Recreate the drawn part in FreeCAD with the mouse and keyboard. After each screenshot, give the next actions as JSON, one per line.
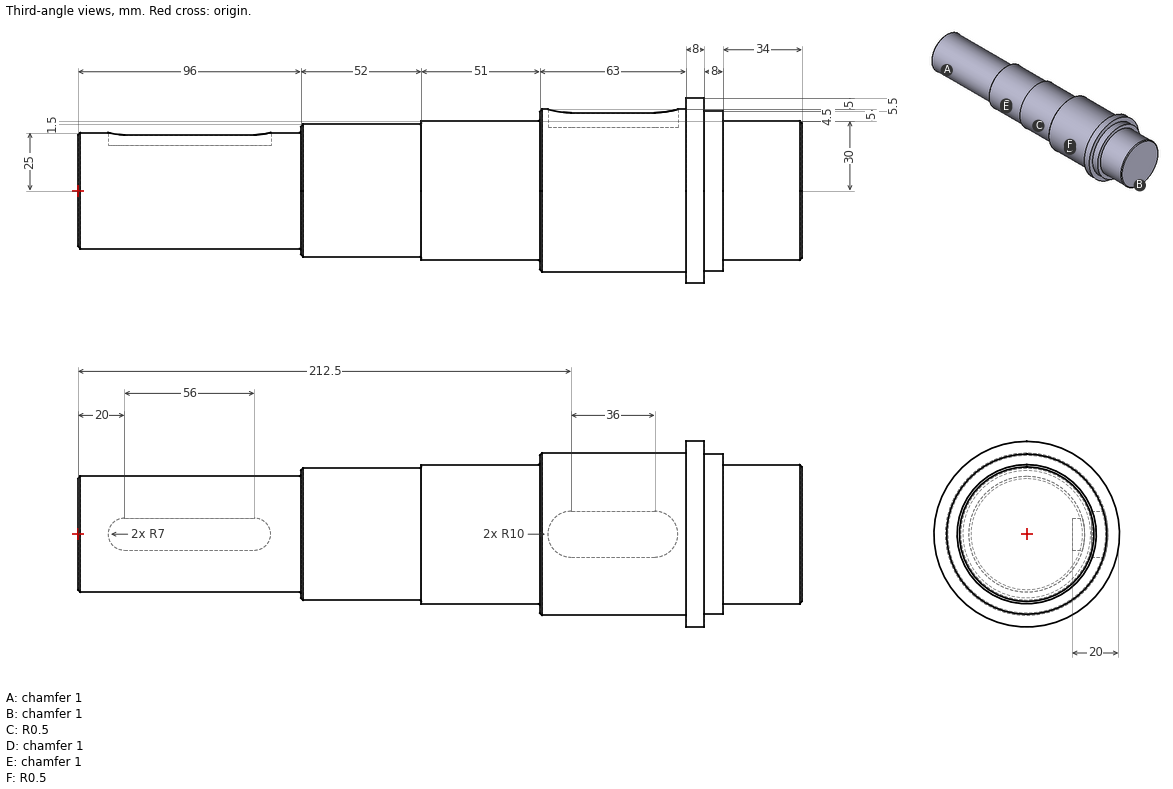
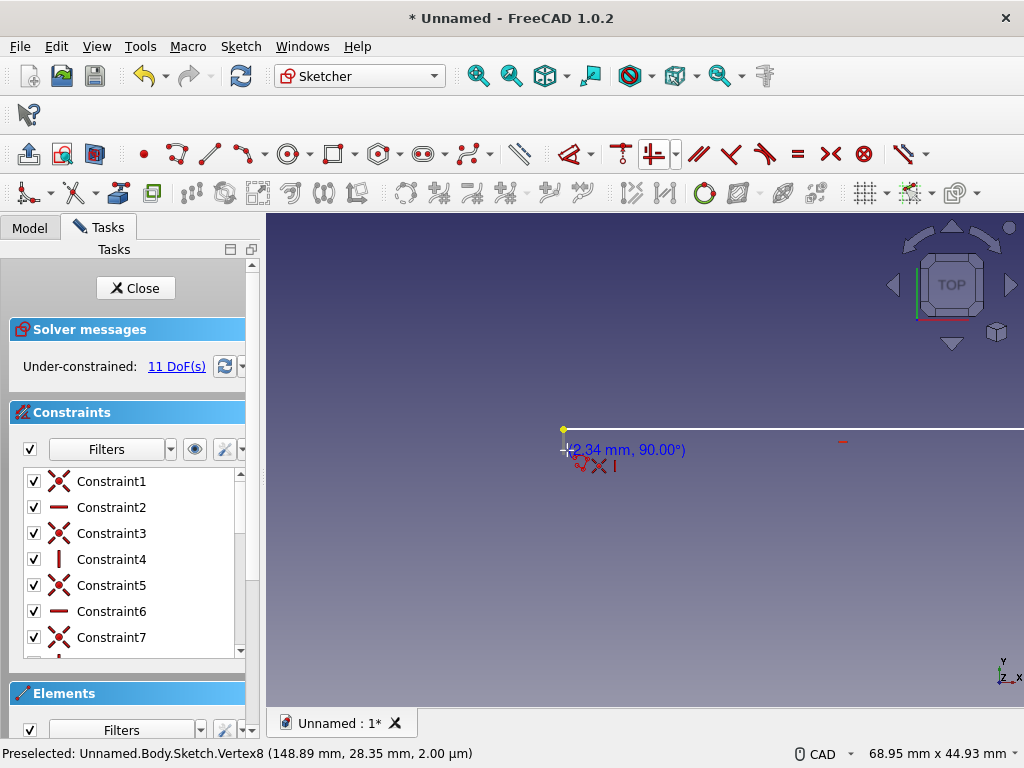
{"action": "left_click", "coordinate": [564, 444]}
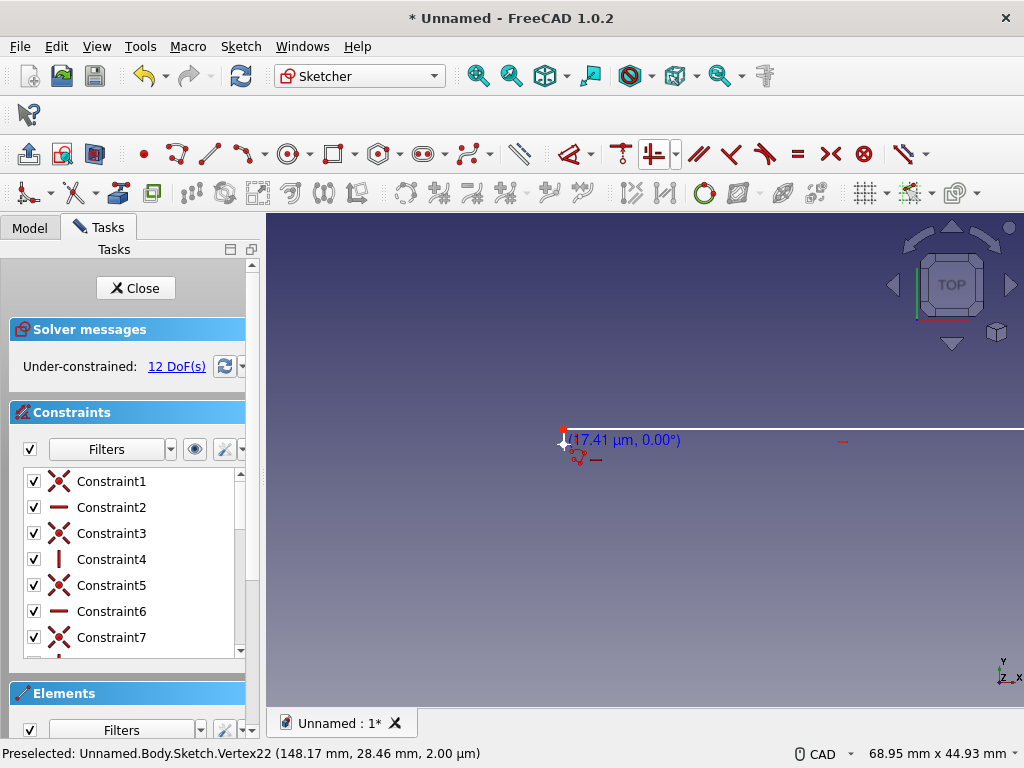
{"action": "scroll", "coordinate": [567, 450], "scroll_direction": "down", "scroll_amount": 11}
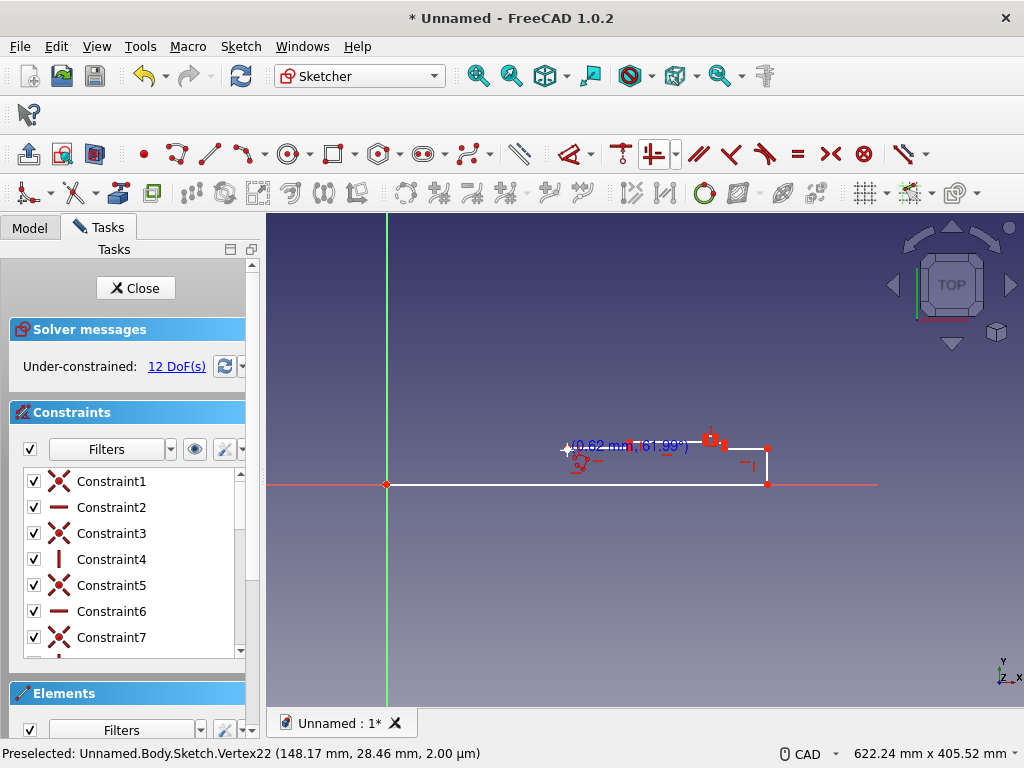
{"action": "left_click", "coordinate": [504, 450]}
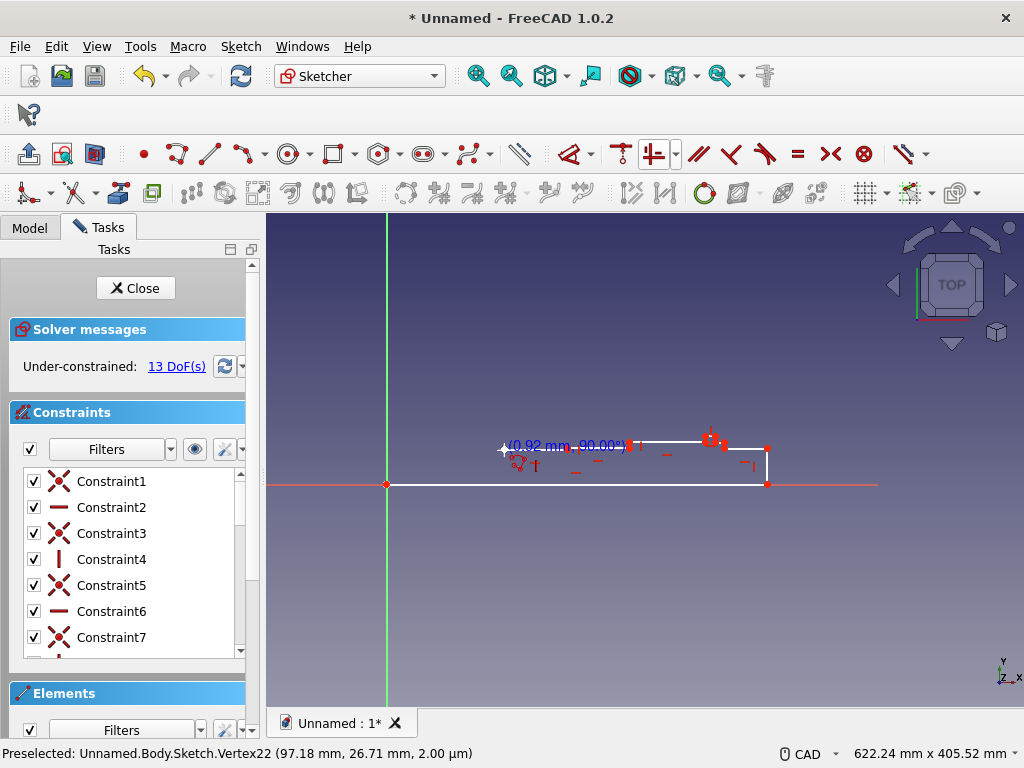
{"action": "scroll", "coordinate": [504, 454], "scroll_direction": "up", "scroll_amount": 7}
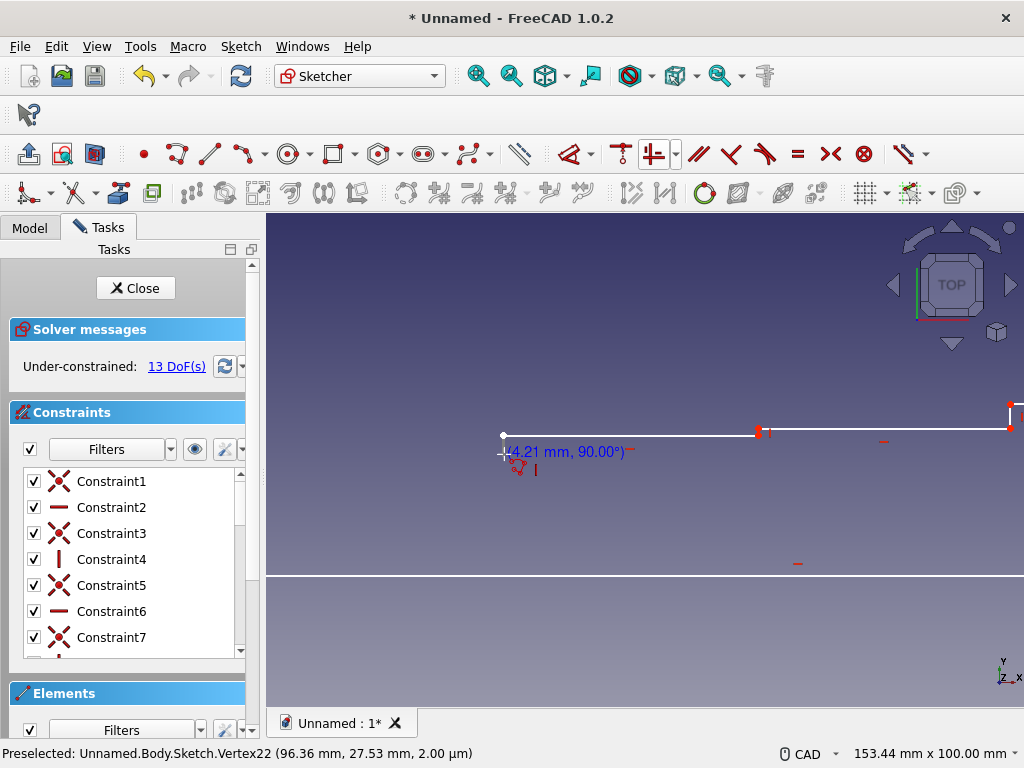
{"action": "left_click", "coordinate": [503, 453]}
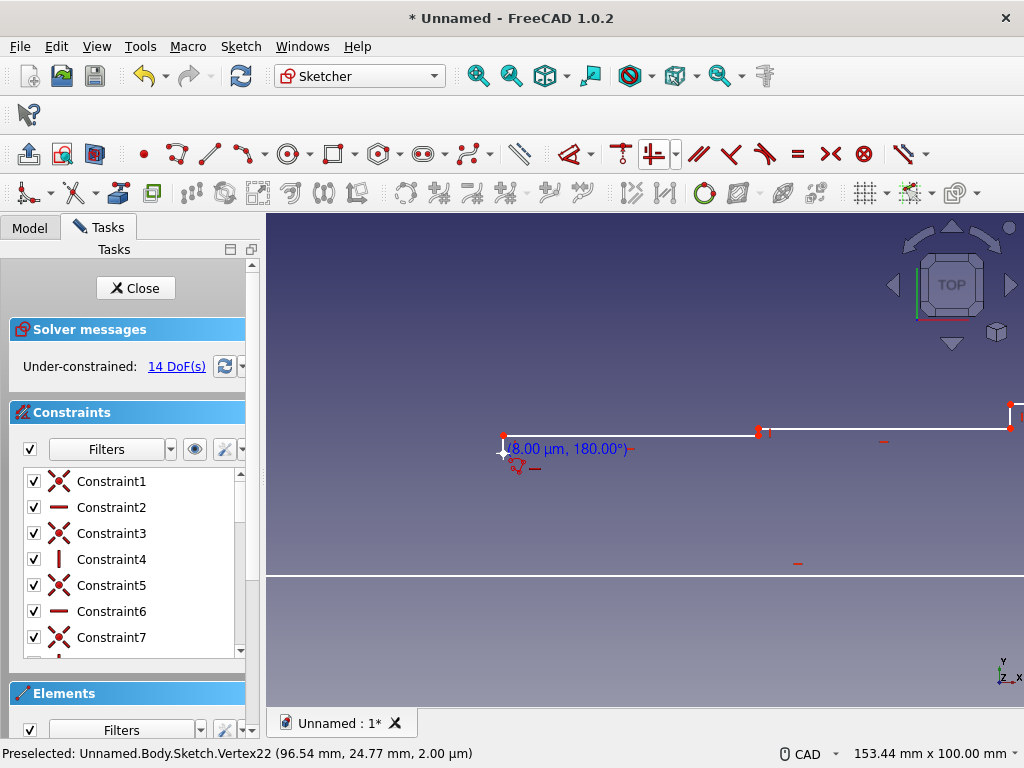
{"action": "scroll", "coordinate": [504, 454], "scroll_direction": "down", "scroll_amount": 7}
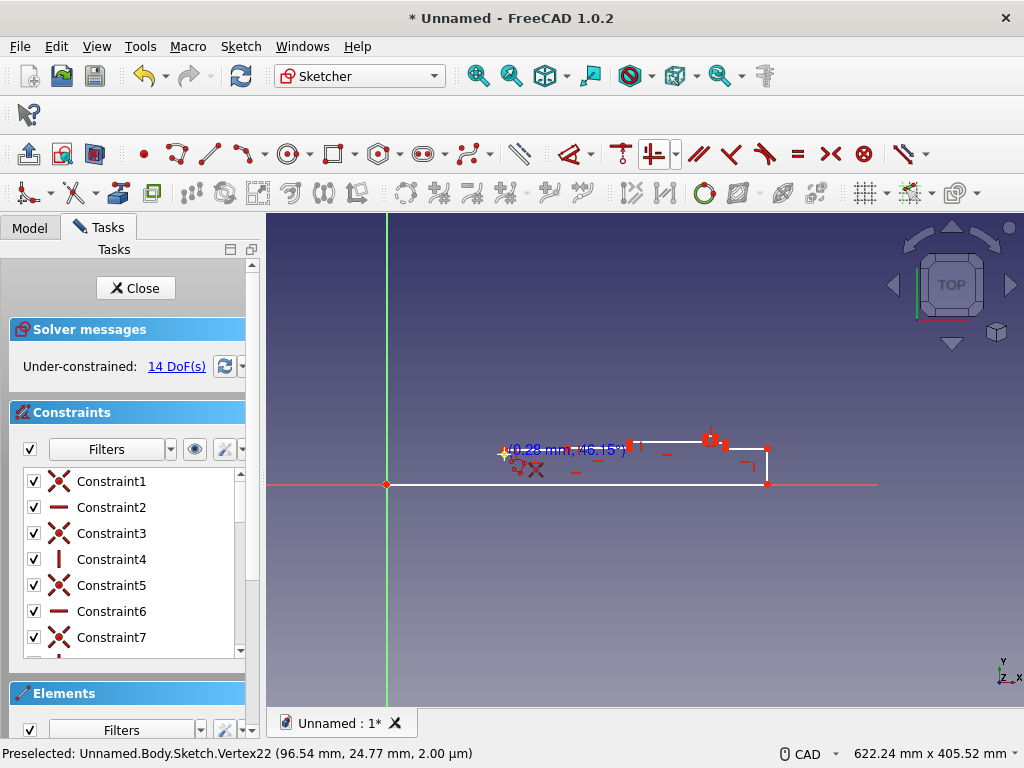
{"action": "left_click", "coordinate": [396, 454]}
{"action": "left_click", "coordinate": [387, 485]}
{"action": "key", "text": "Escape"}
{"action": "key", "text": "Escape"}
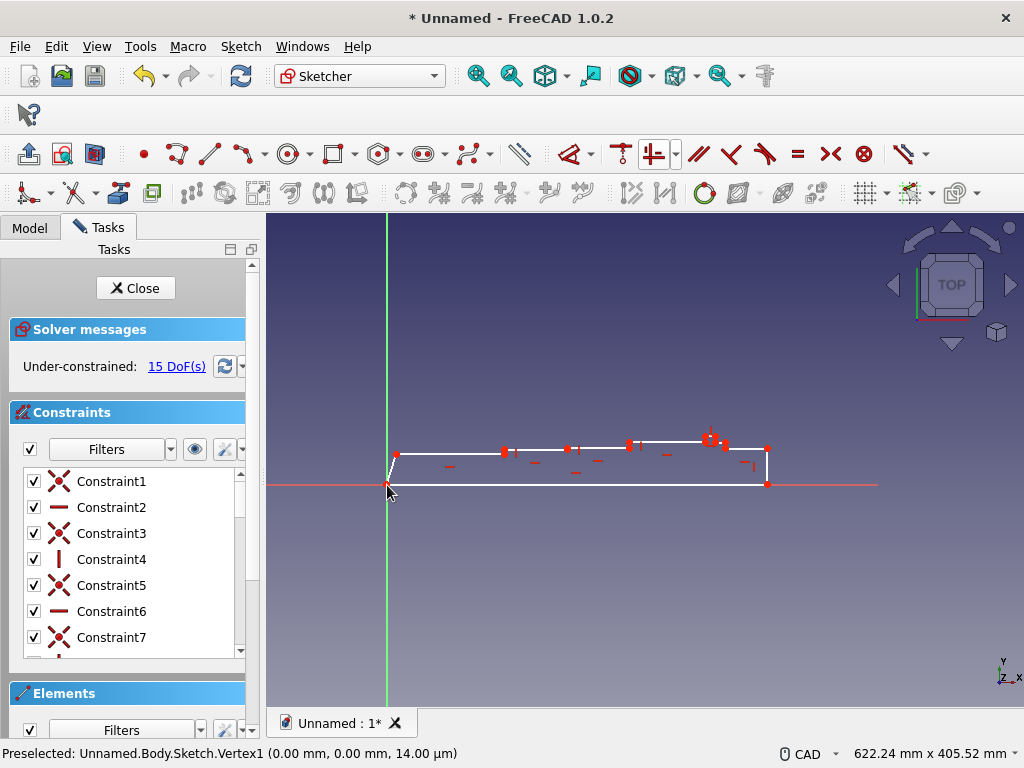
{"action": "scroll", "coordinate": [389, 475], "scroll_direction": "up", "scroll_amount": 3}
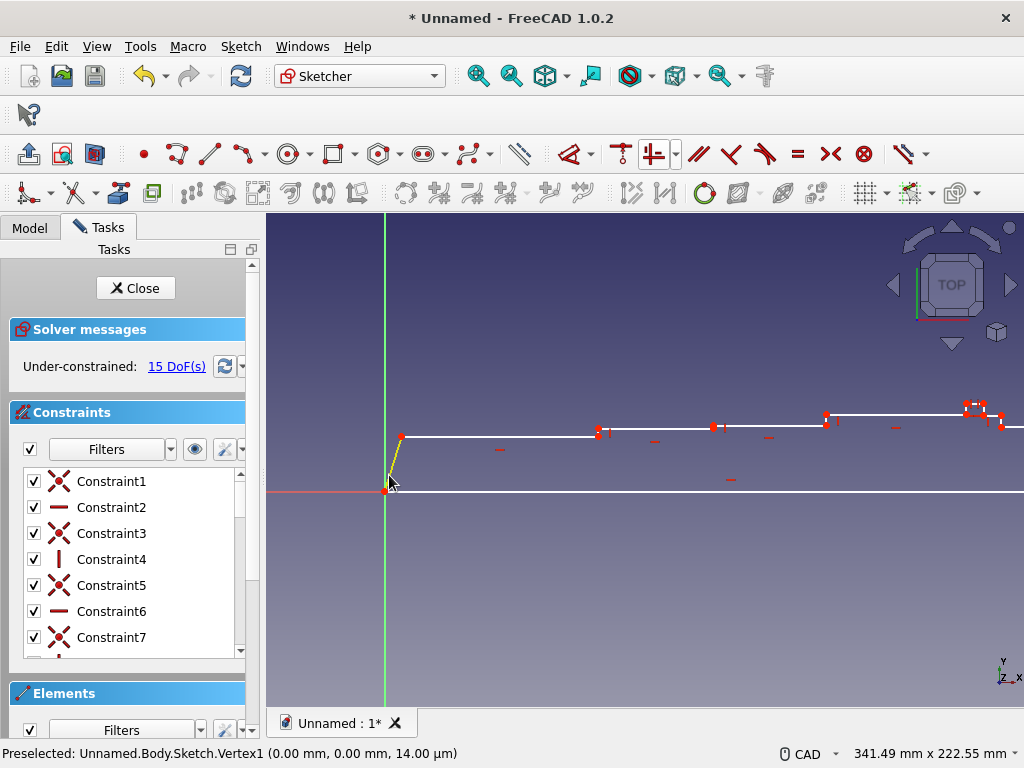
{"action": "left_click", "coordinate": [390, 475]}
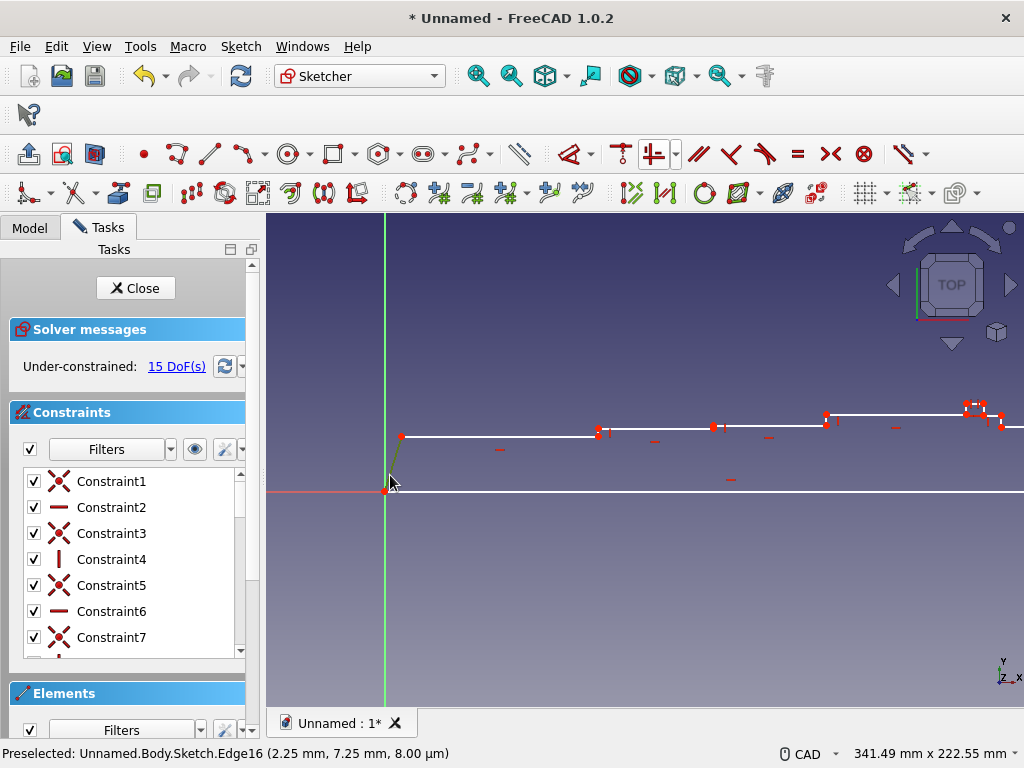
{"action": "key", "text": "v"}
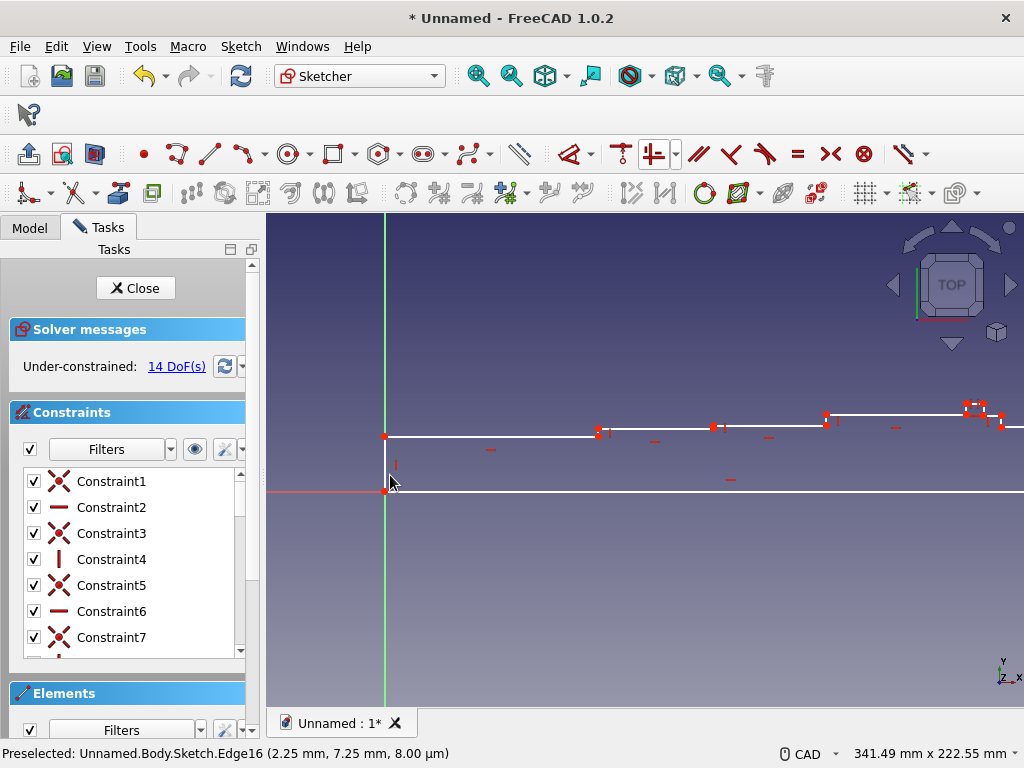
{"action": "scroll", "coordinate": [389, 475], "scroll_direction": "down", "scroll_amount": 3}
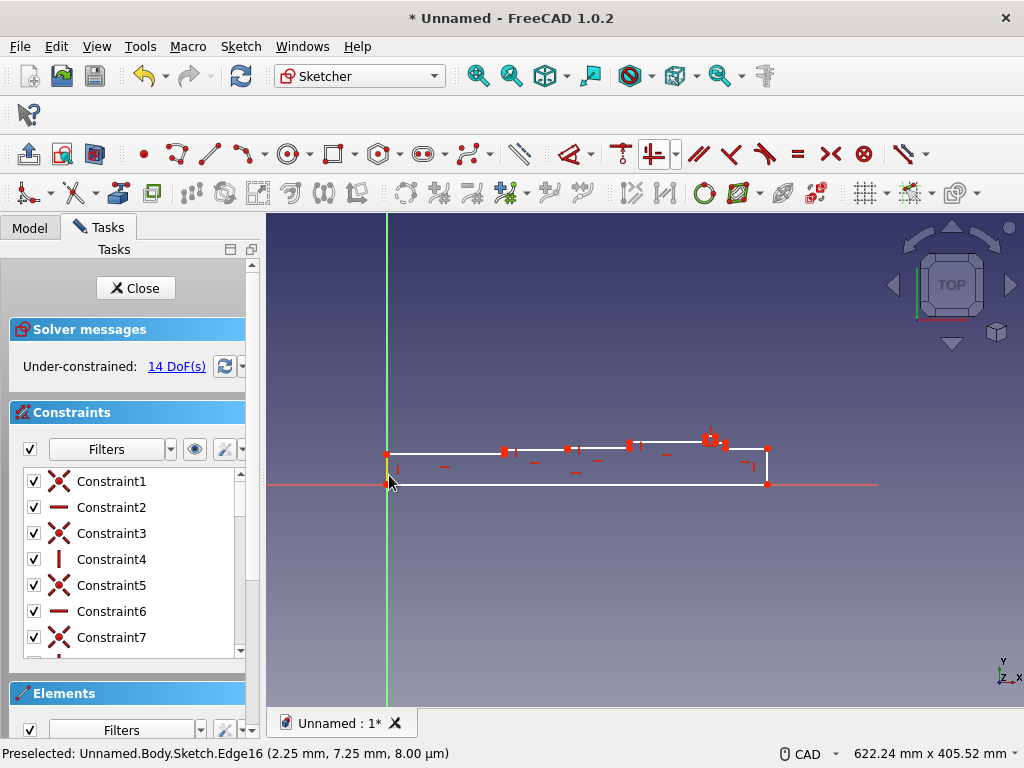
{"action": "scroll", "coordinate": [720, 443], "scroll_direction": "up", "scroll_amount": 8}